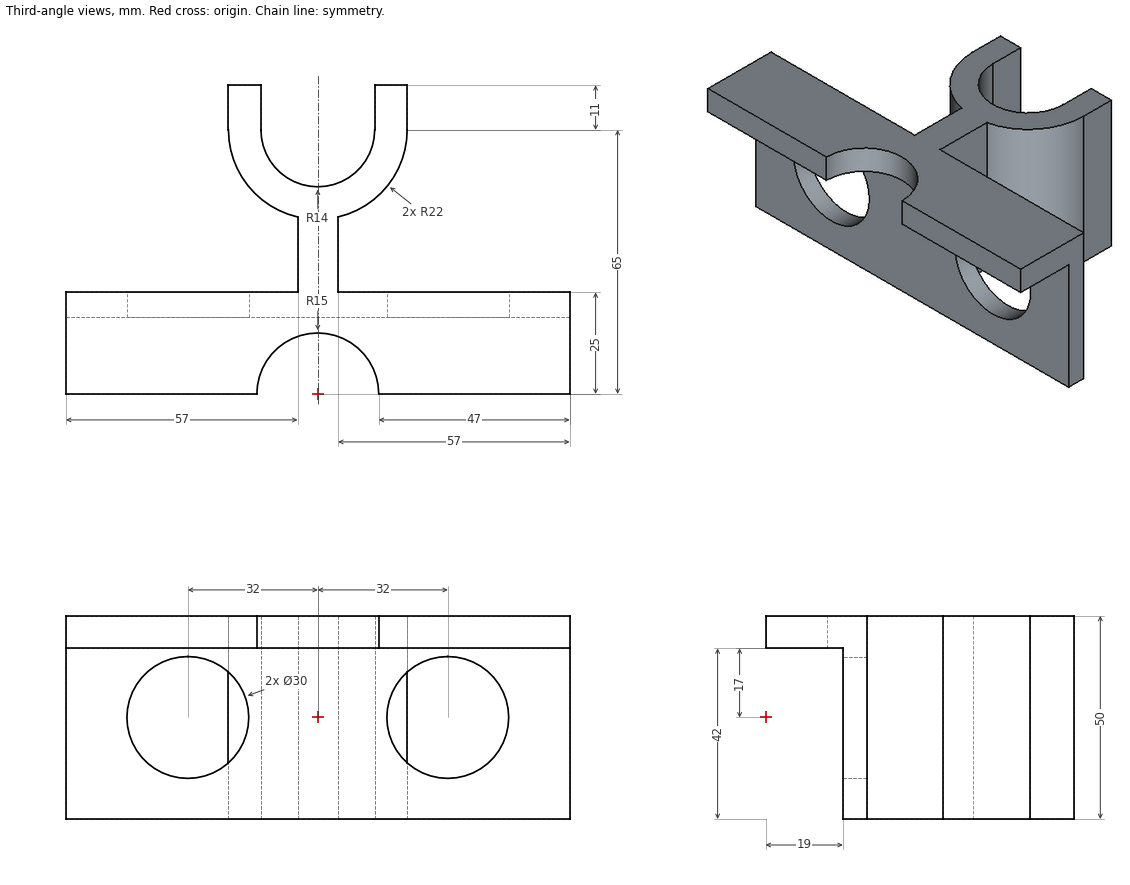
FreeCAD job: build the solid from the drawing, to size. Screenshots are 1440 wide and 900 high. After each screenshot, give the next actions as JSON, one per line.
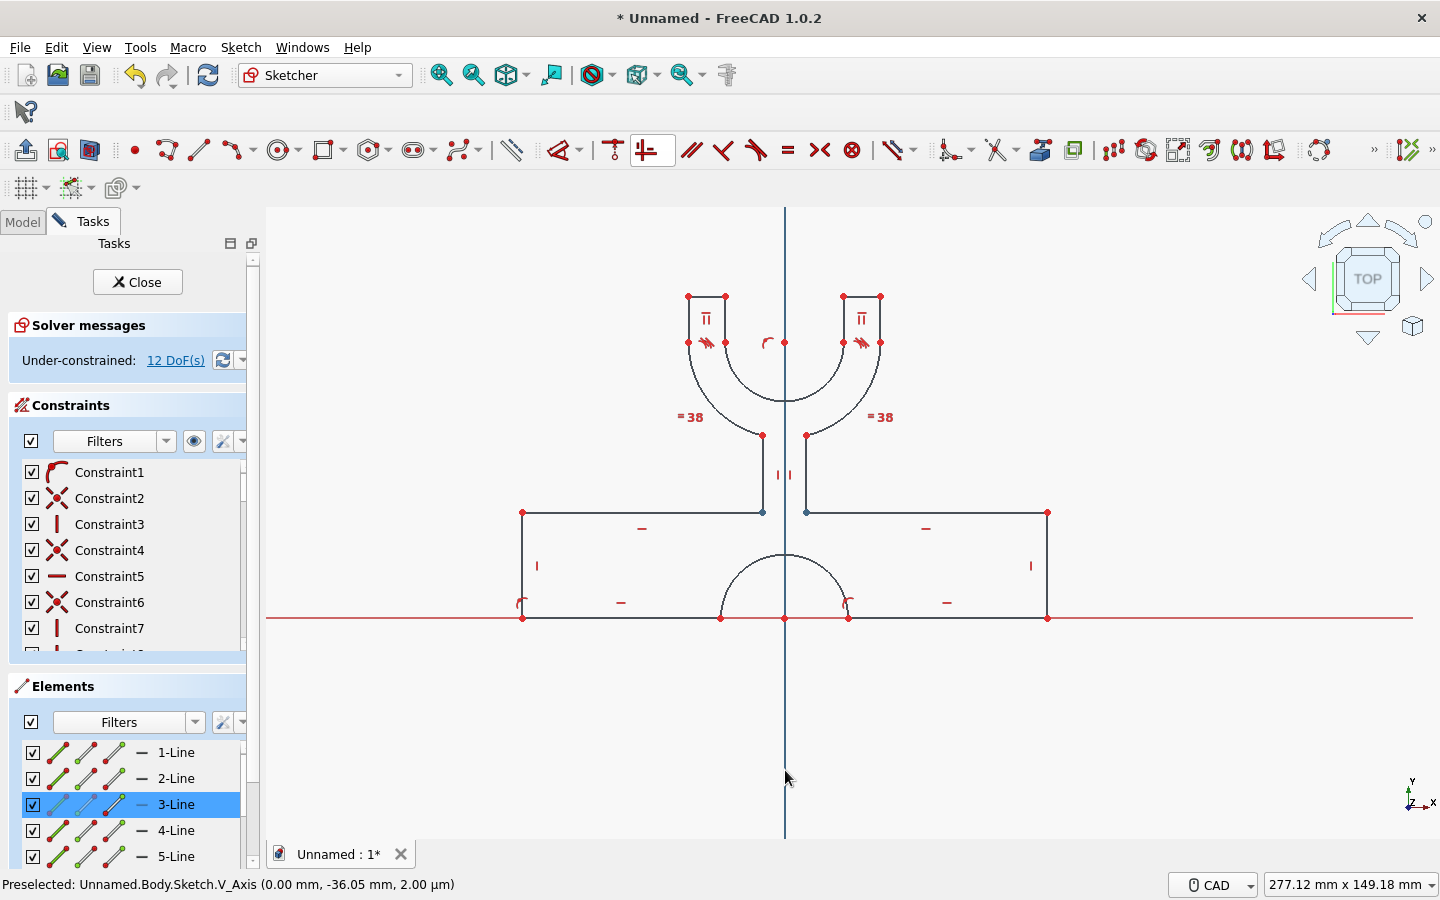
{"action": "left_click", "coordinate": [820, 150]}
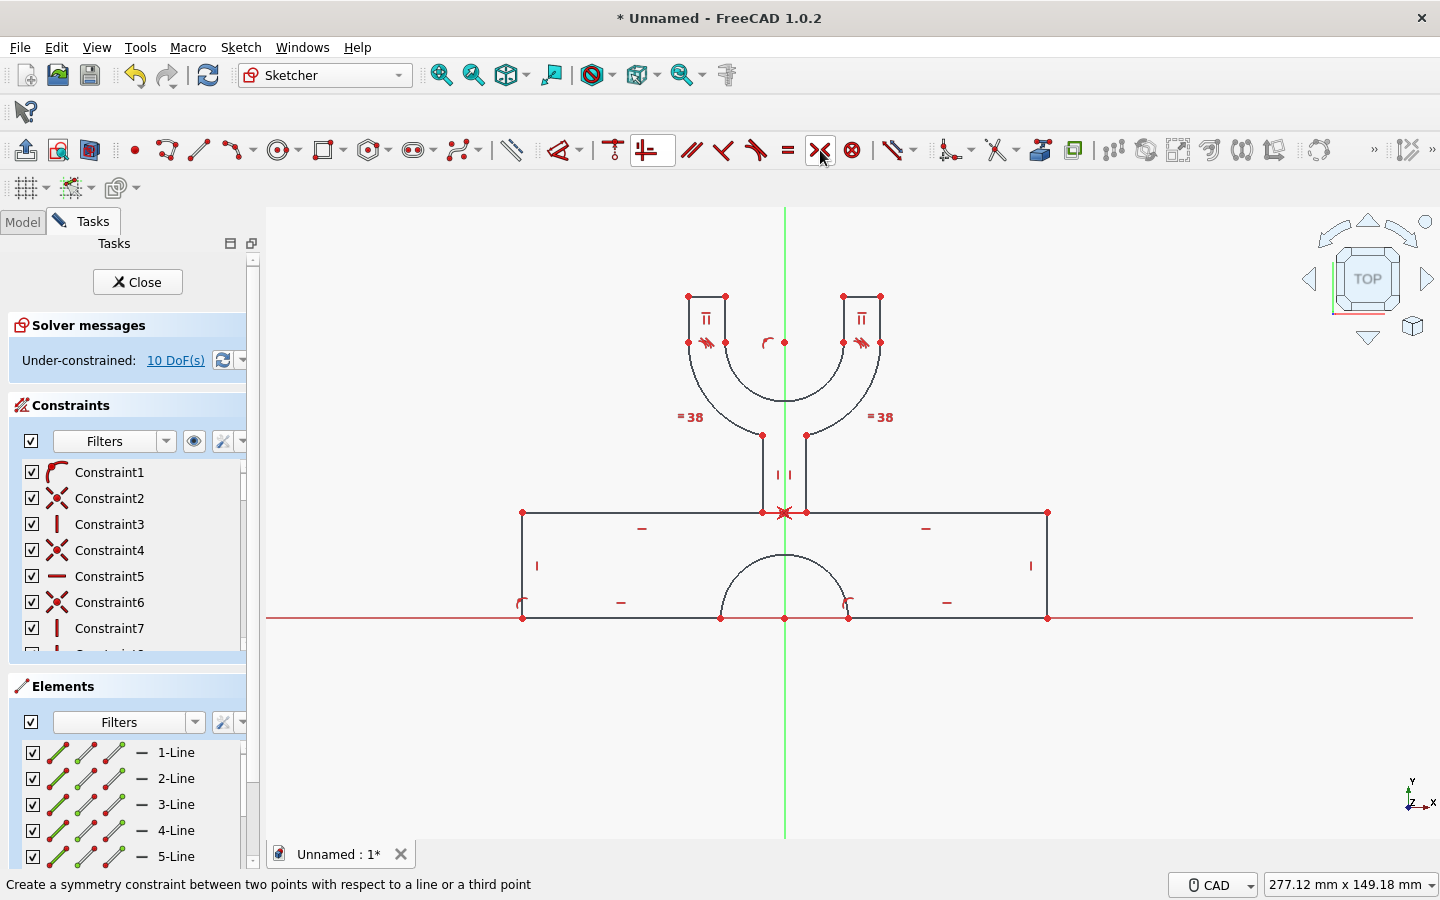
{"action": "left_click", "coordinate": [558, 150]}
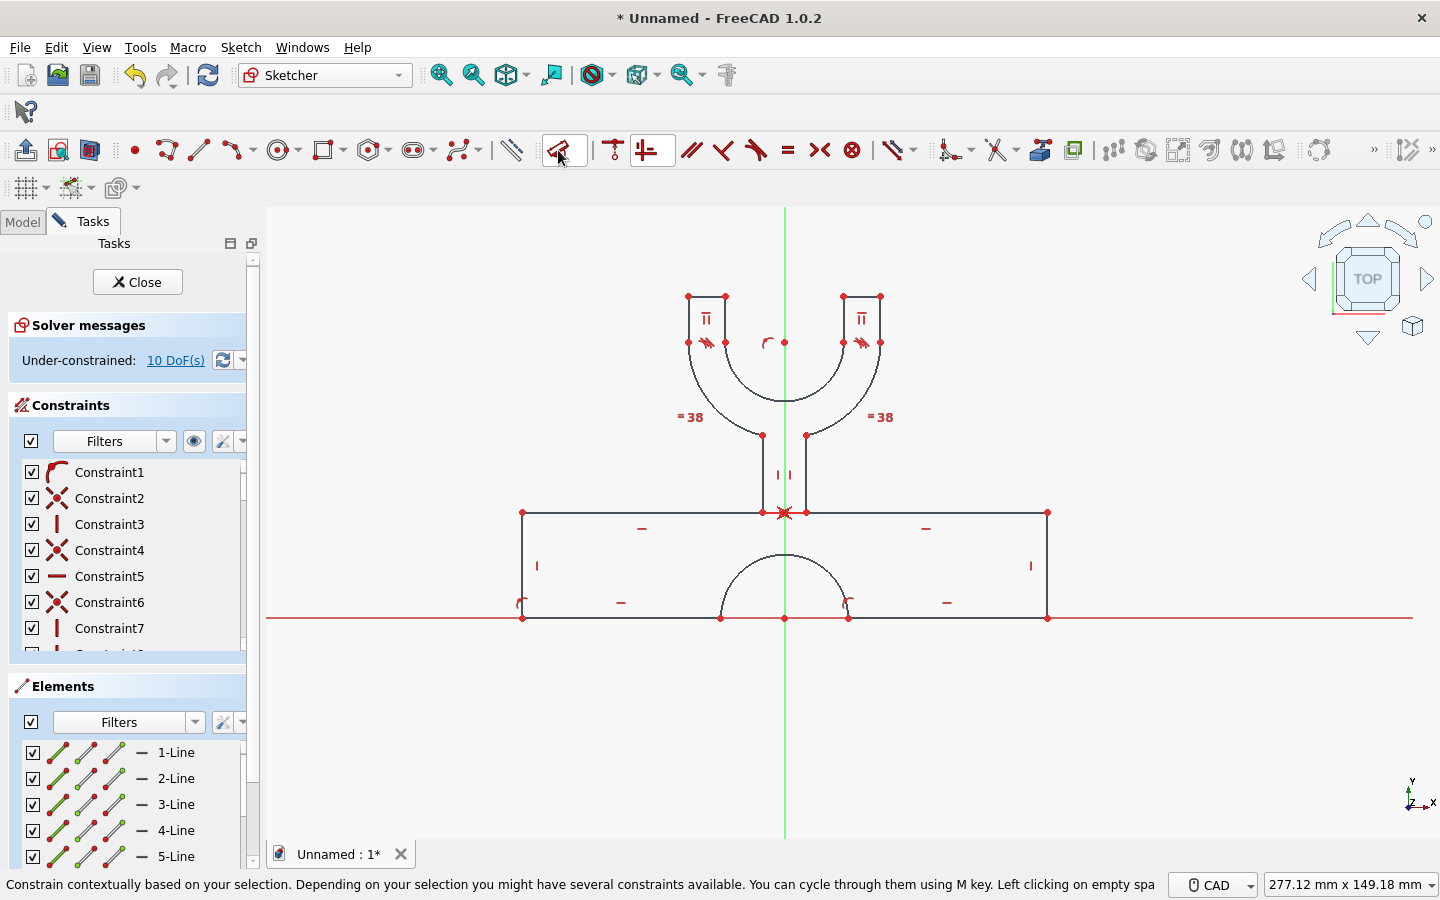
{"action": "left_click", "coordinate": [841, 420]}
{"action": "left_click", "coordinate": [860, 446]}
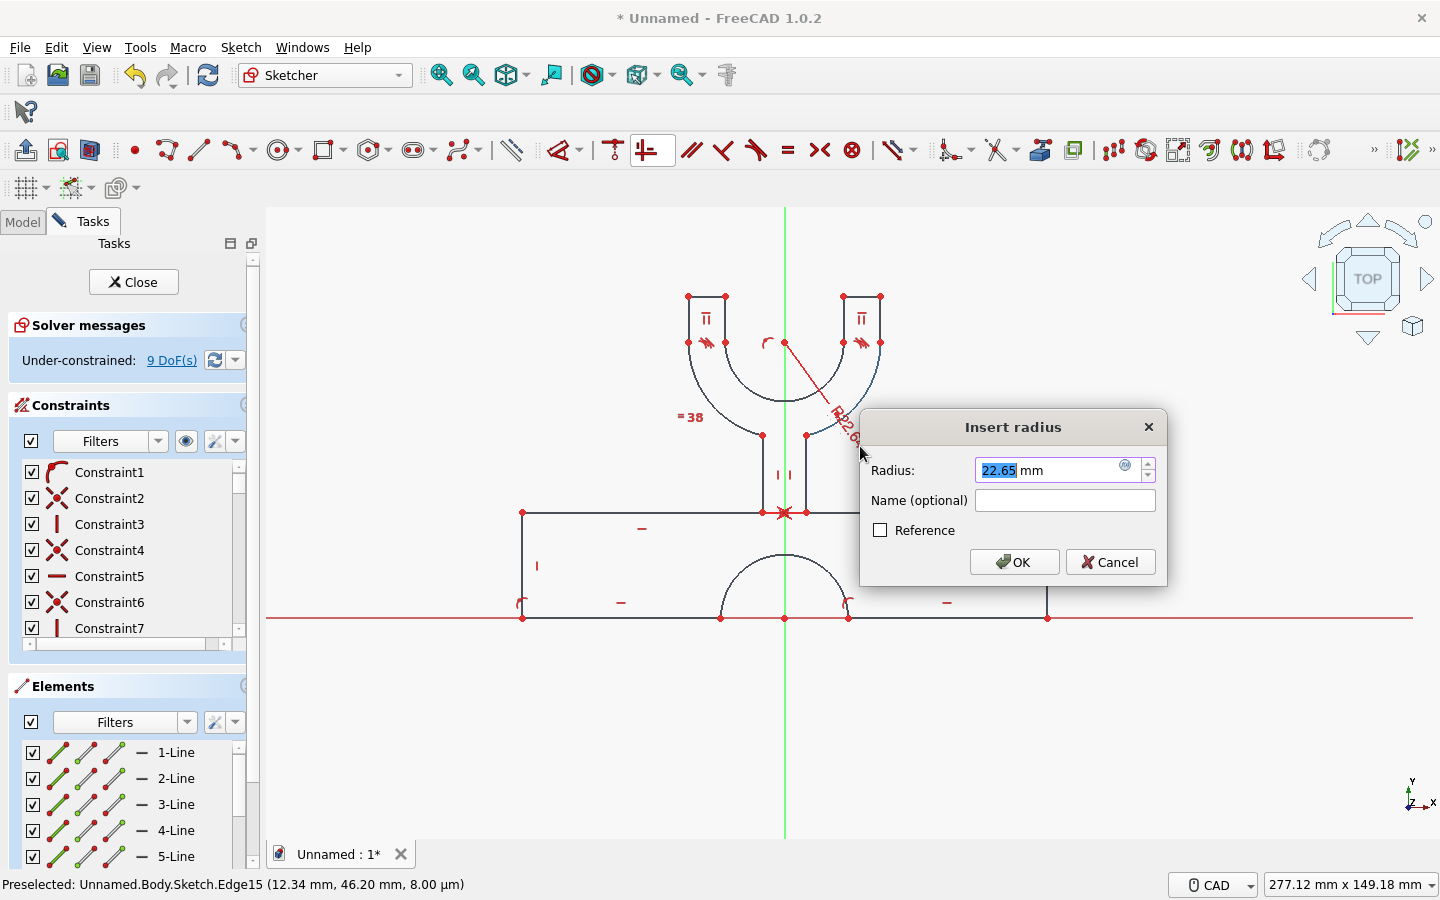
{"action": "type", "text": "22"}
{"action": "key", "text": "Return"}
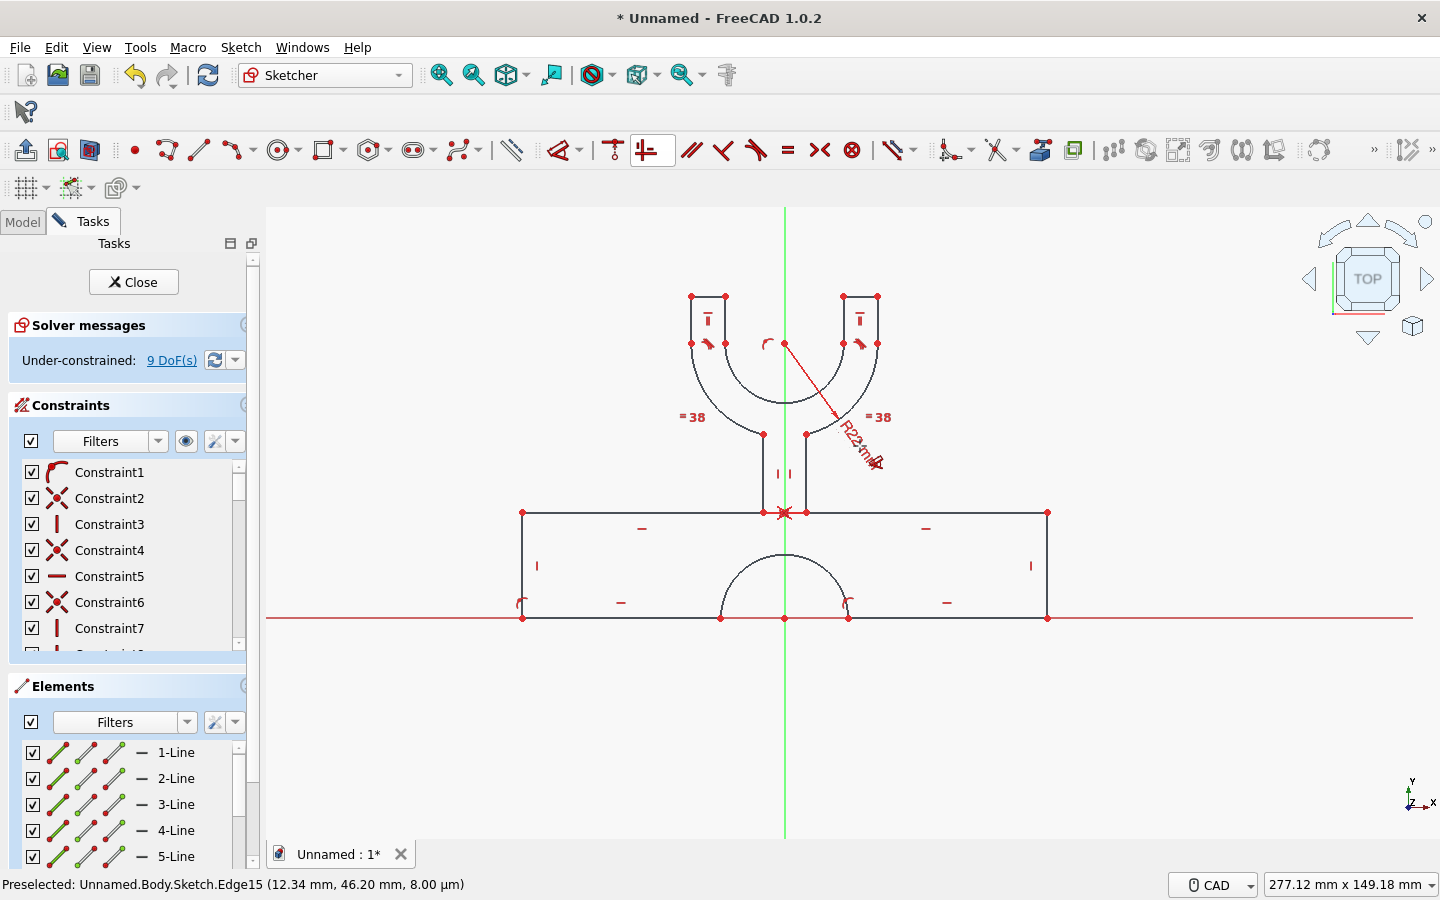
{"action": "left_click", "coordinate": [750, 392]}
{"action": "left_click", "coordinate": [838, 270]}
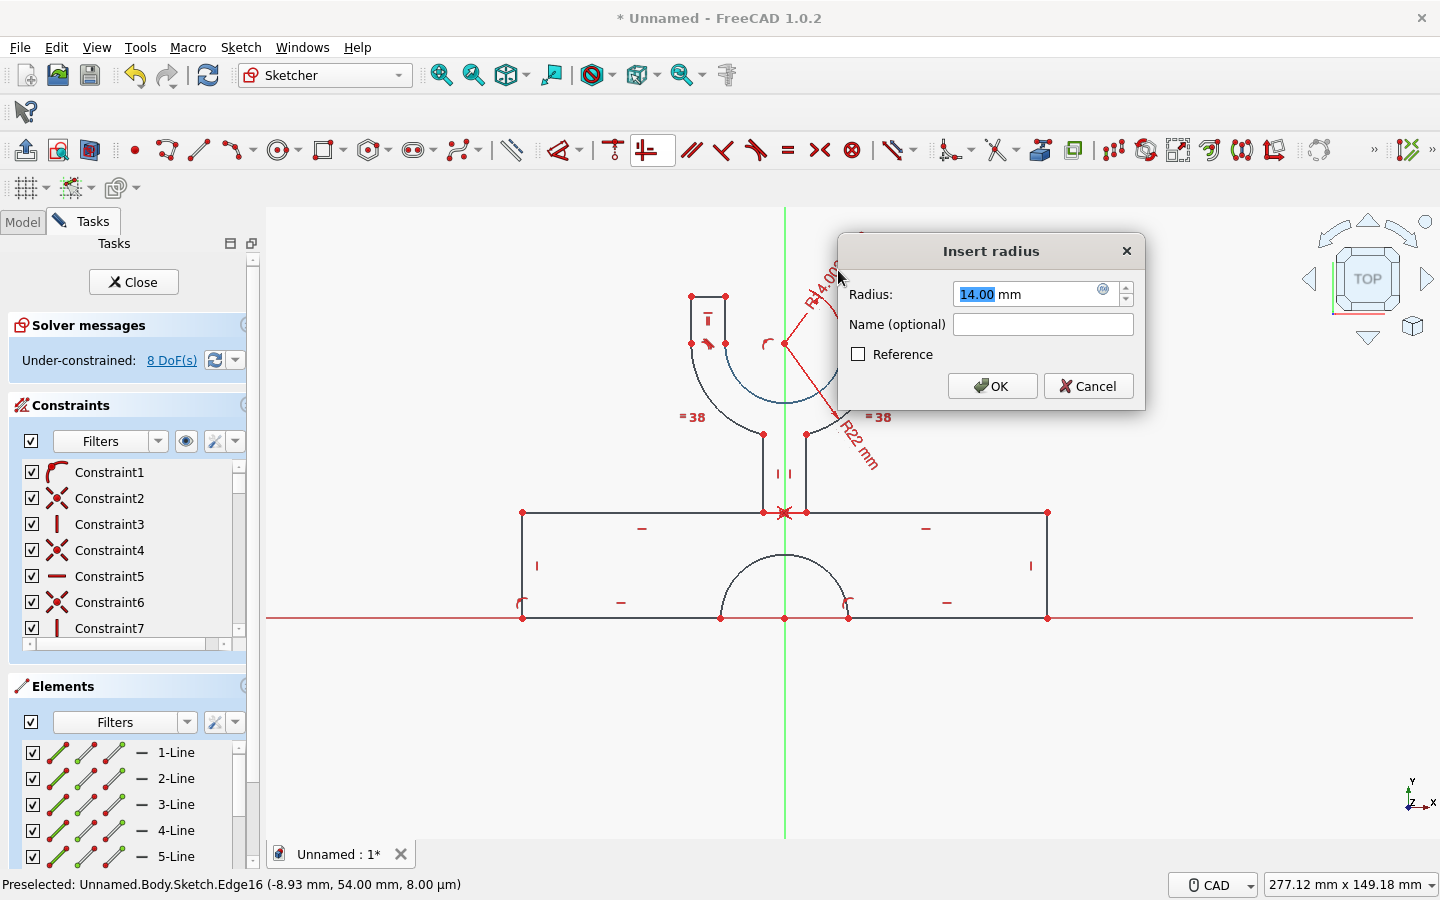
{"action": "type", "text": "14"}
{"action": "key", "text": "Return"}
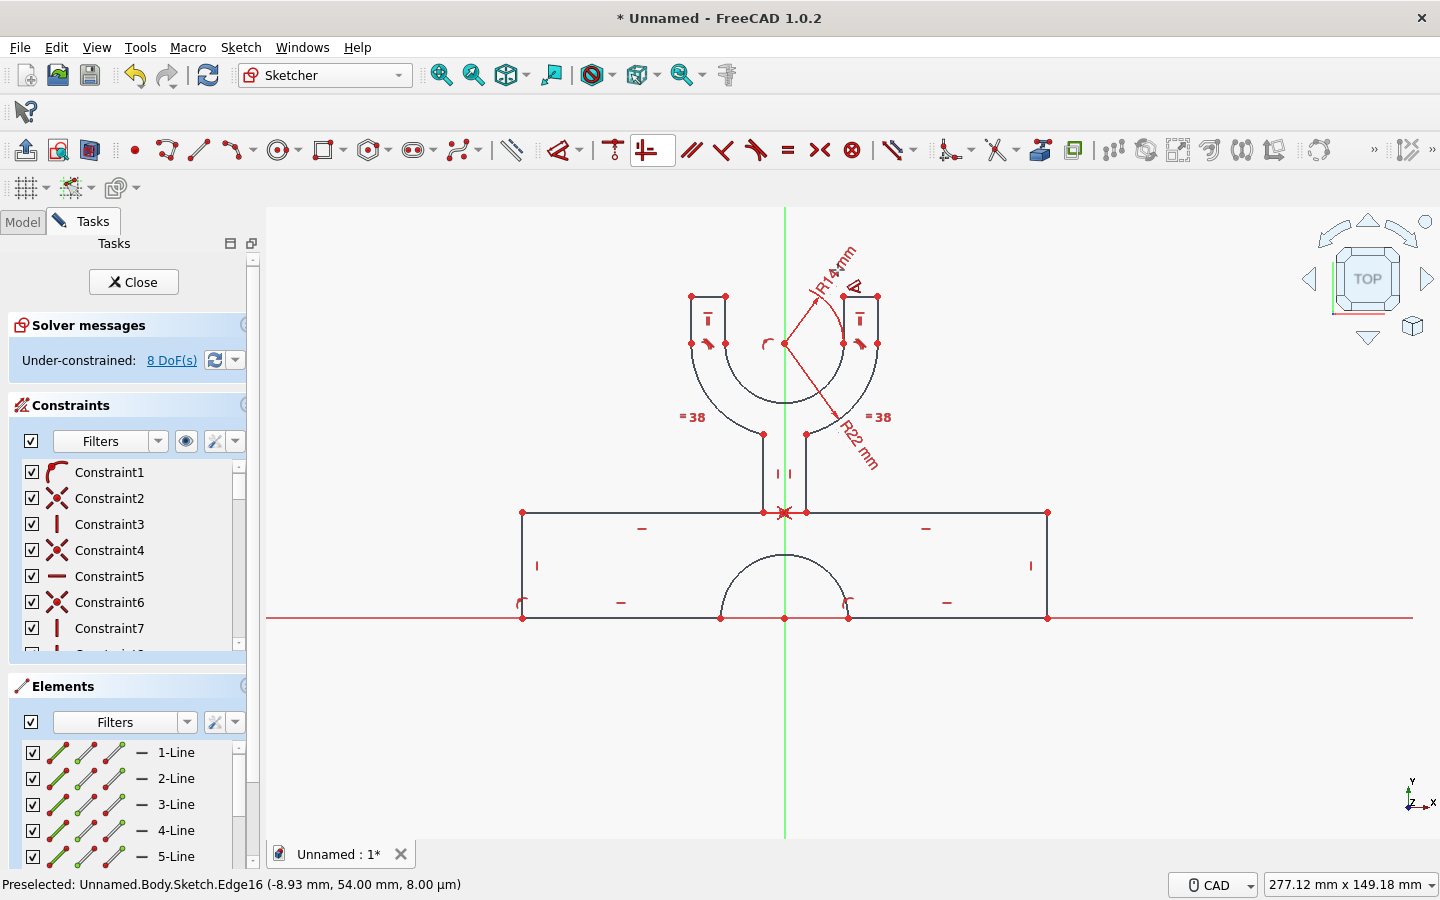
{"action": "left_click", "coordinate": [822, 567]}
{"action": "left_click", "coordinate": [841, 541]}